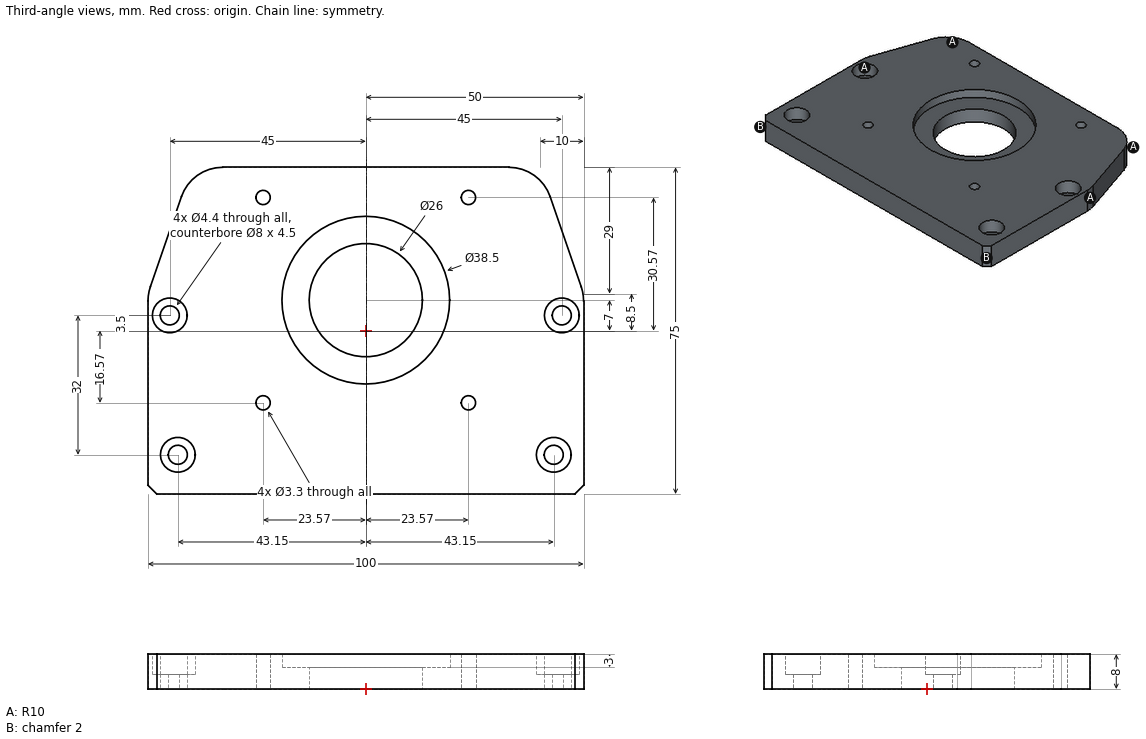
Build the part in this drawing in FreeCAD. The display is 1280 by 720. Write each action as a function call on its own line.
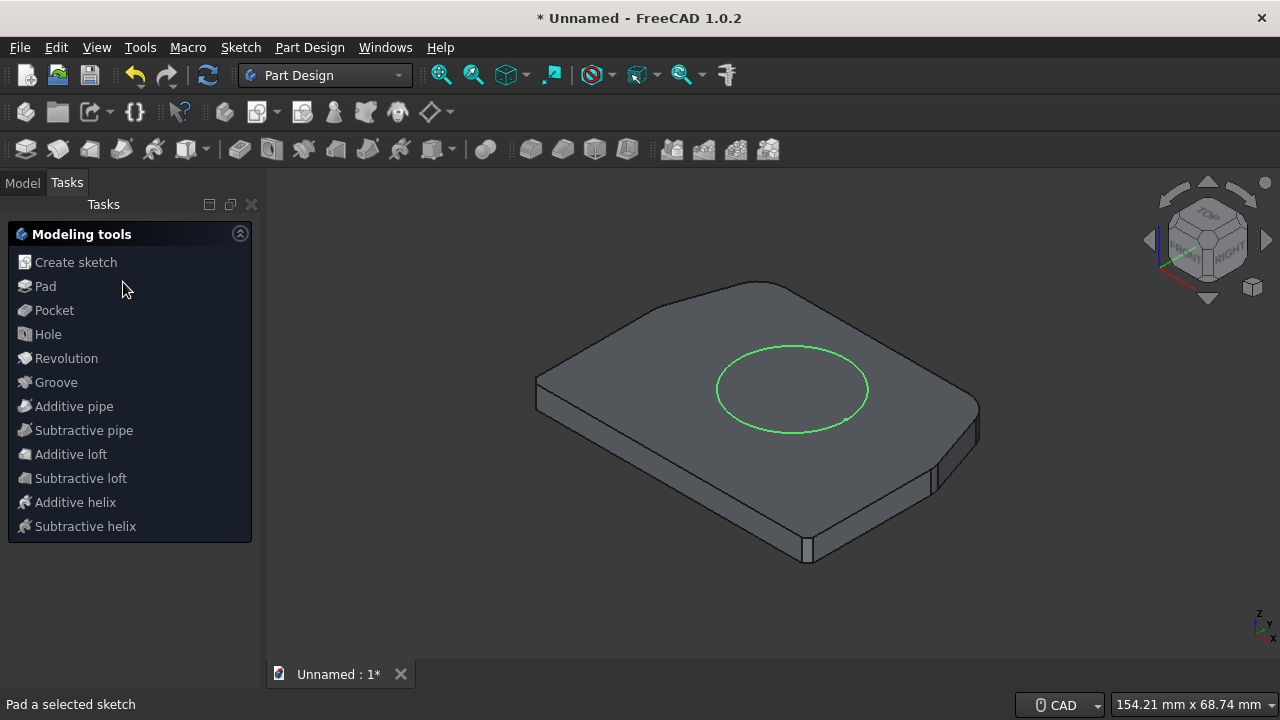
click(240, 150)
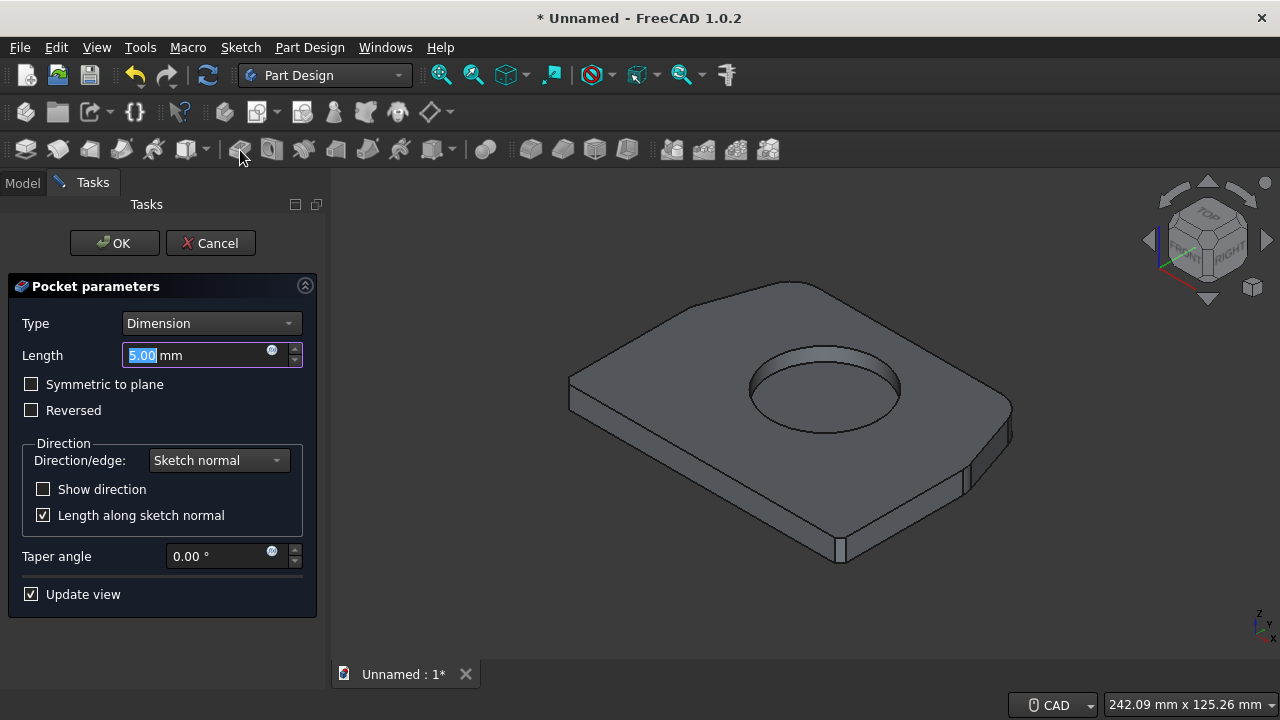
text(3)
key(Tab)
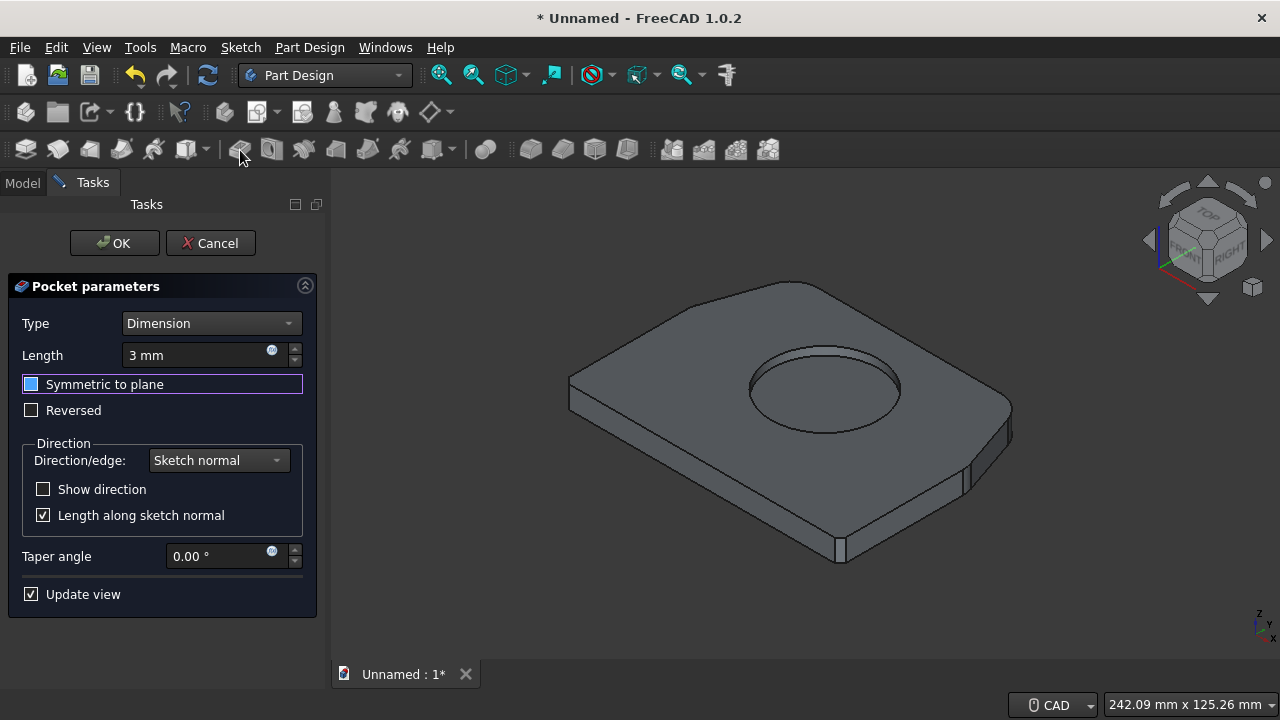
click(115, 243)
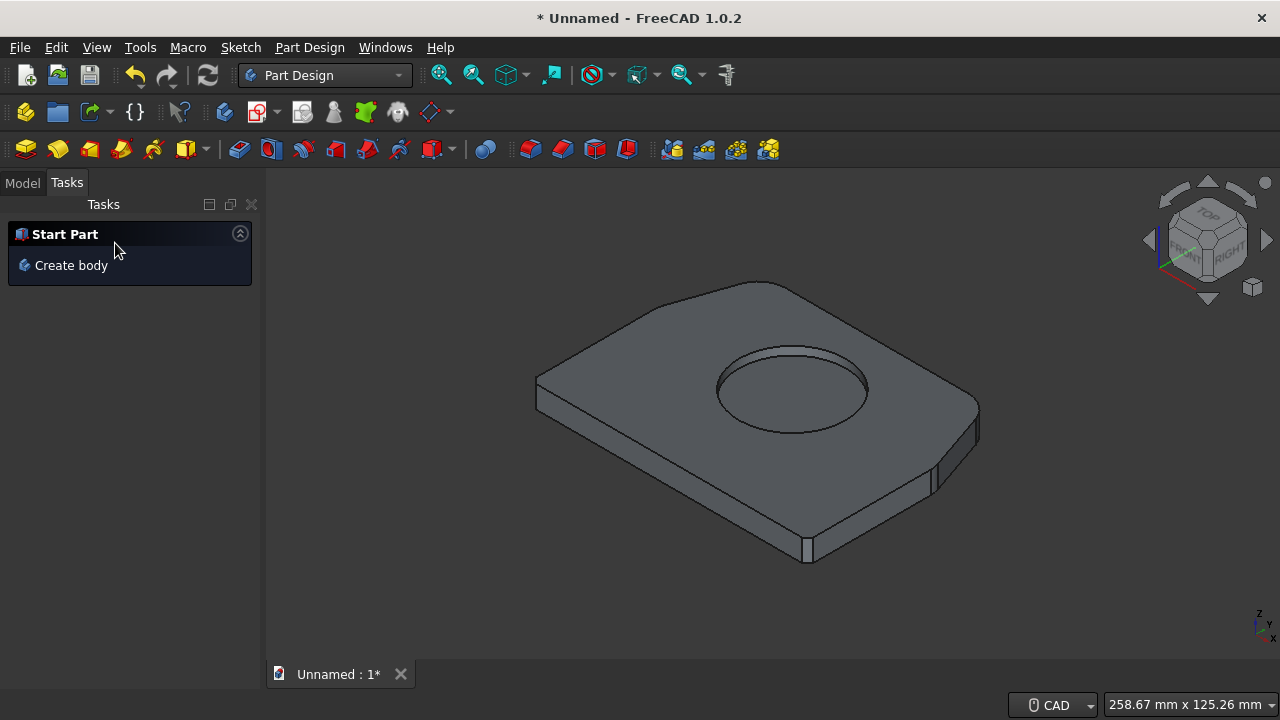
click(792, 398)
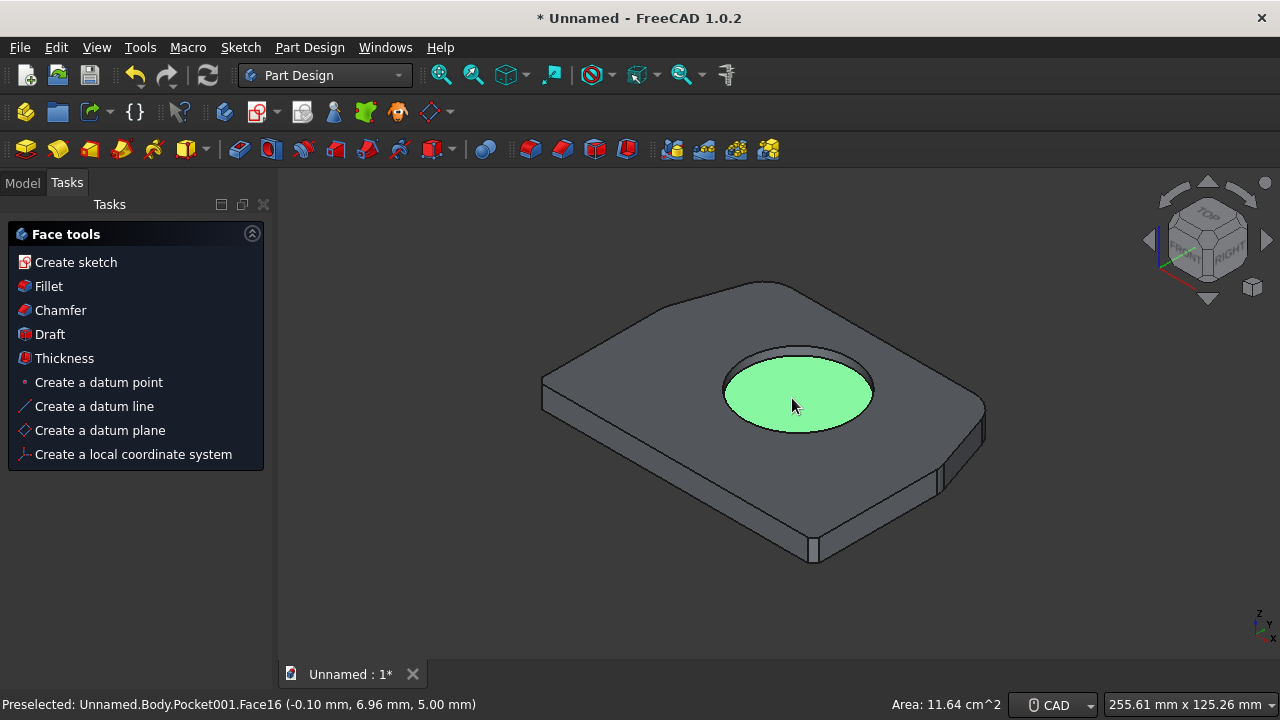
click(258, 112)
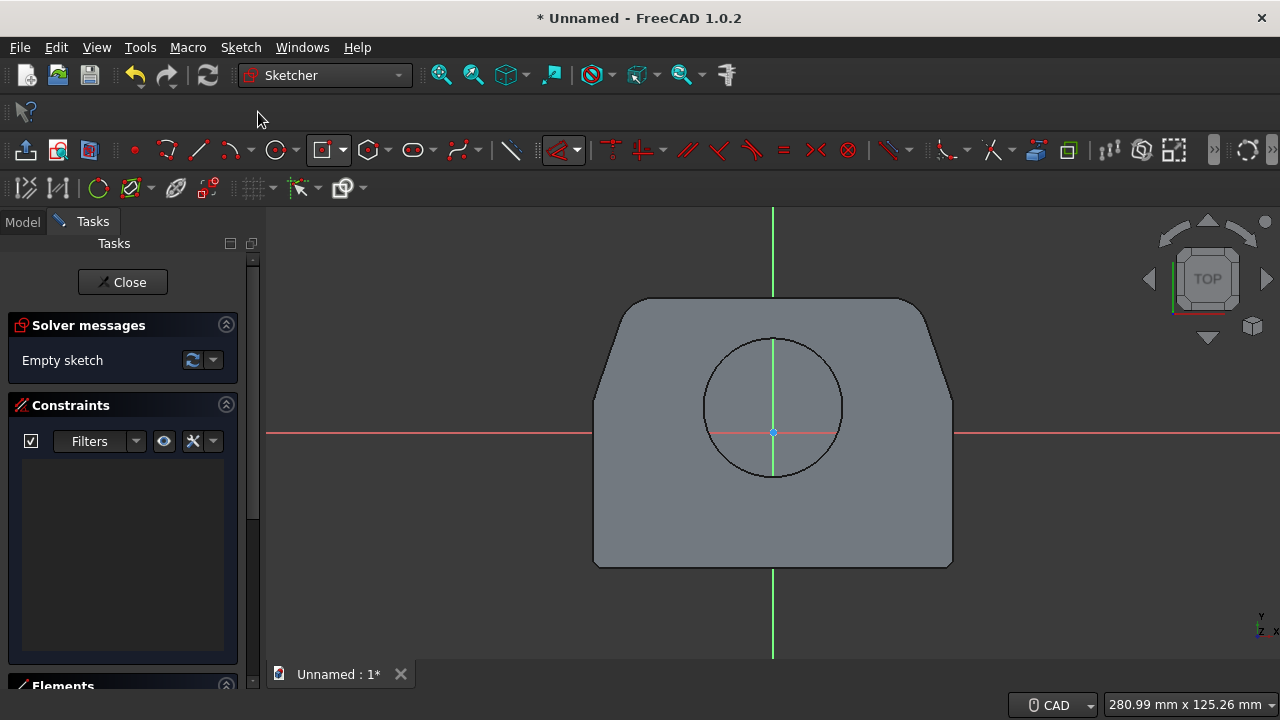
scroll(813, 393, up, 5)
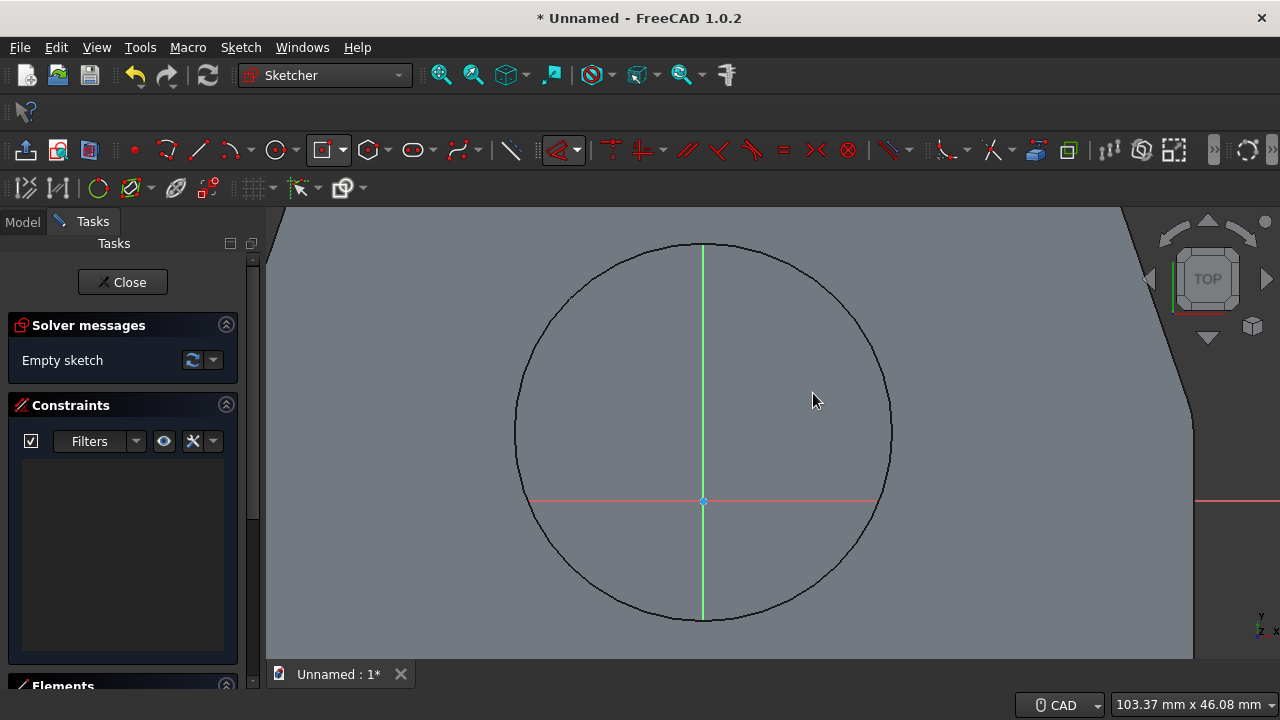
key(g)
key(c)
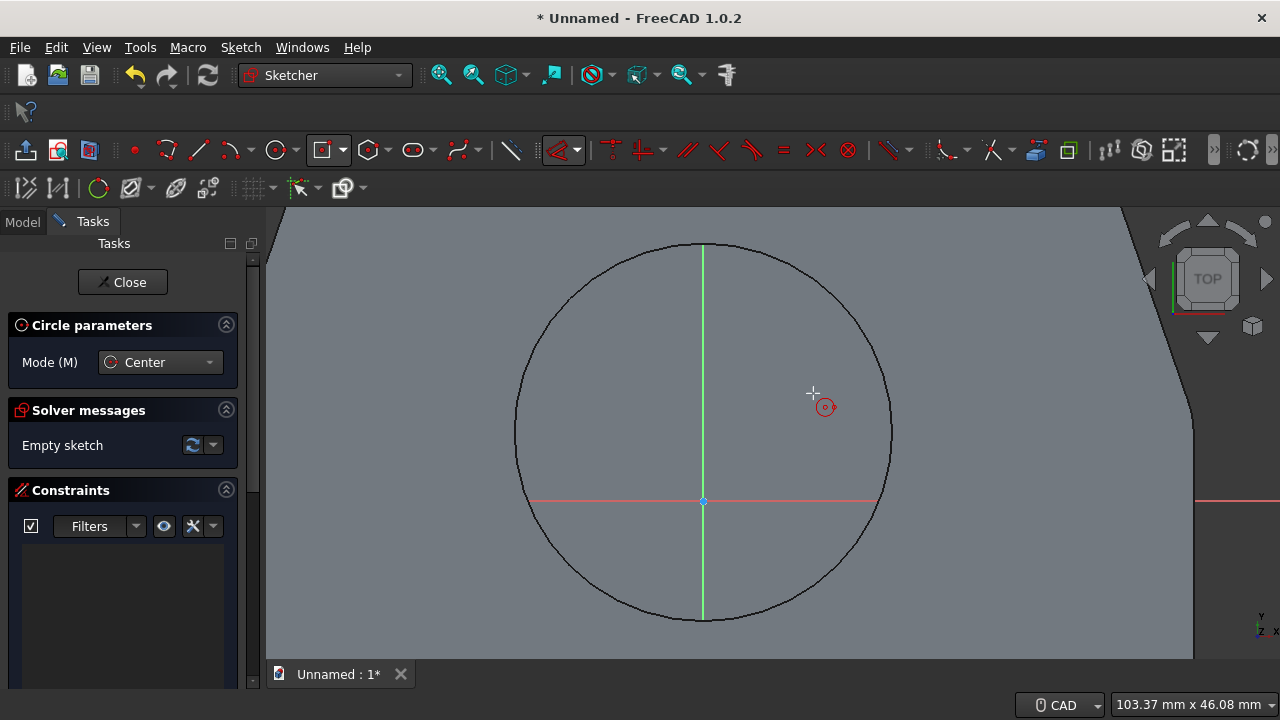
click(703, 432)
click(794, 342)
key(Escape)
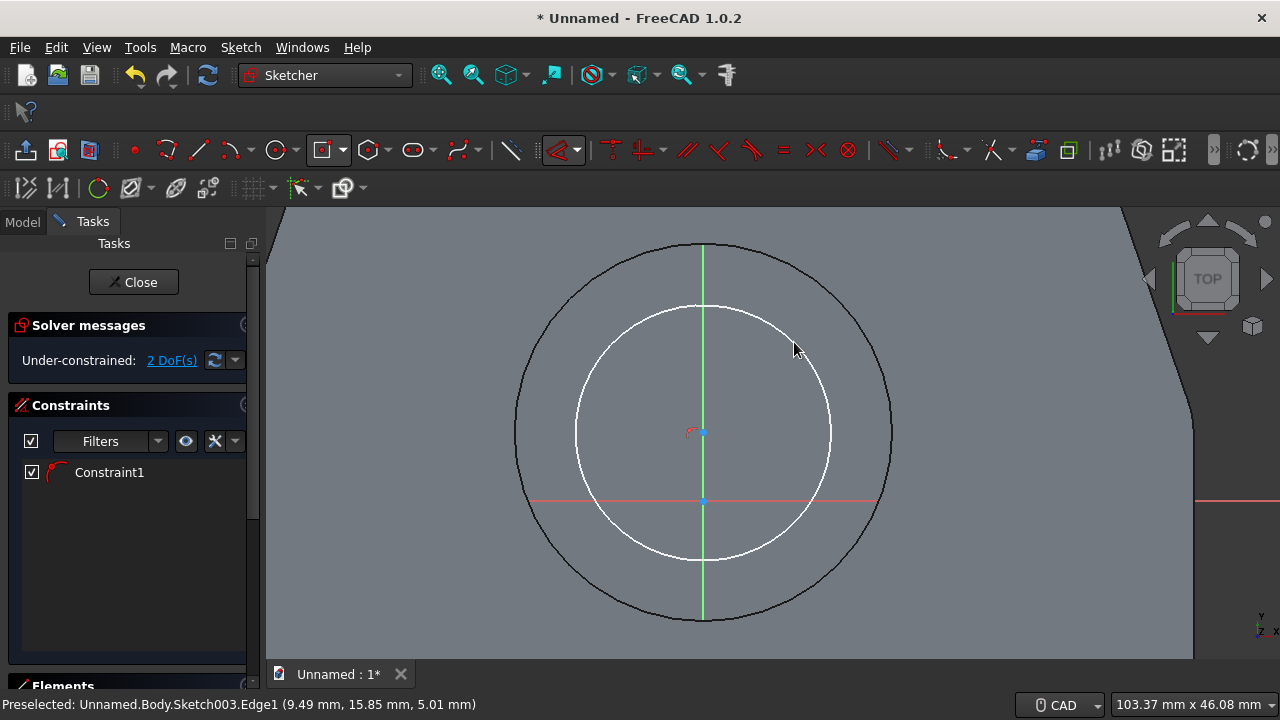
click(793, 342)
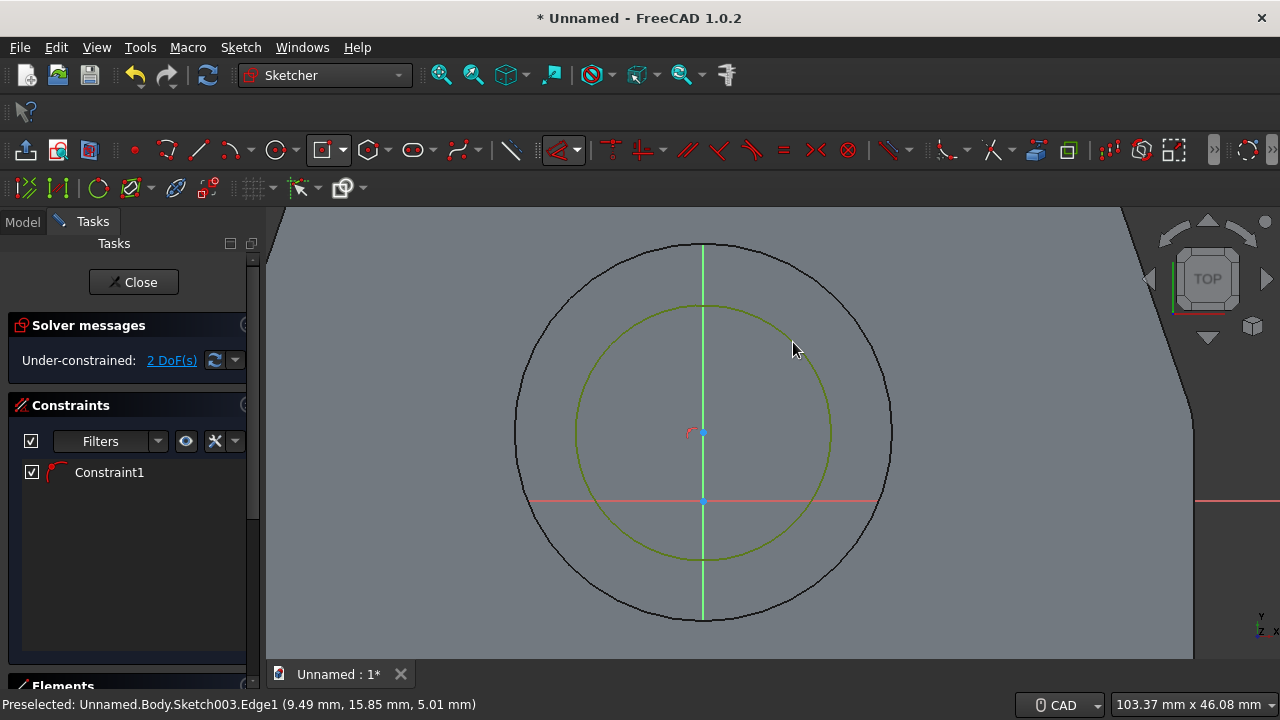
key(k)
key(o)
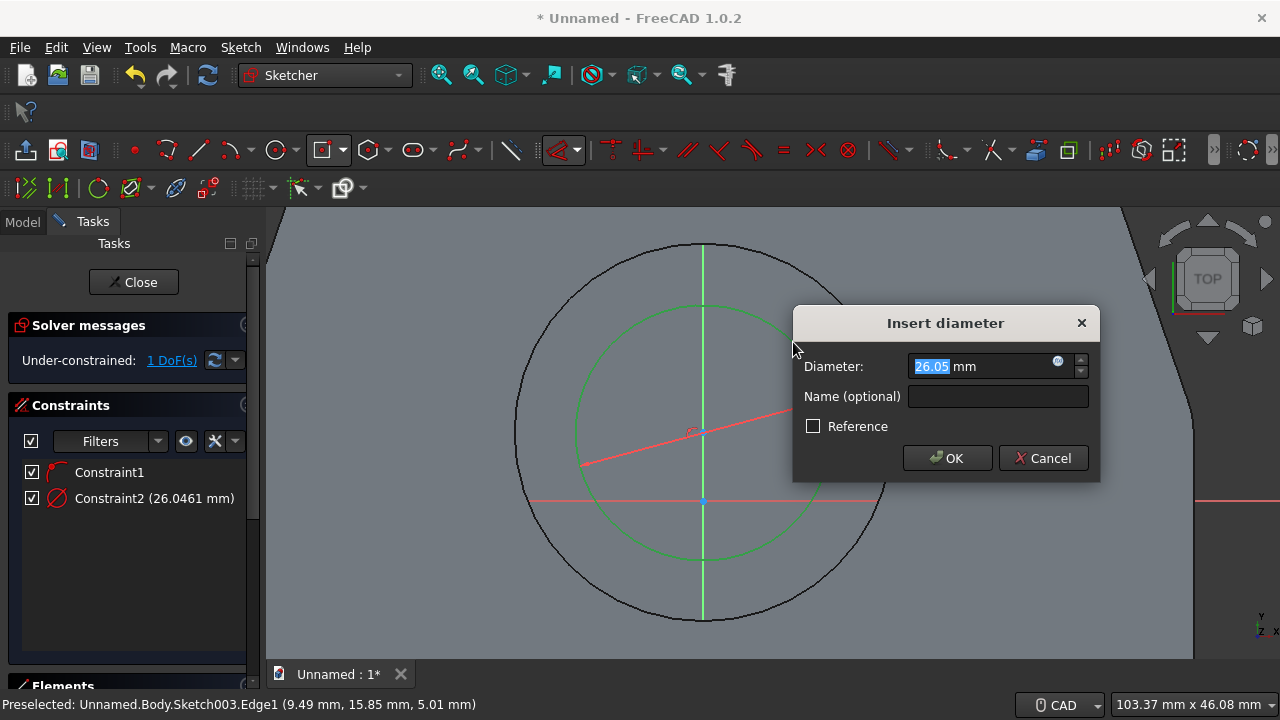
text(26)
key(Return)